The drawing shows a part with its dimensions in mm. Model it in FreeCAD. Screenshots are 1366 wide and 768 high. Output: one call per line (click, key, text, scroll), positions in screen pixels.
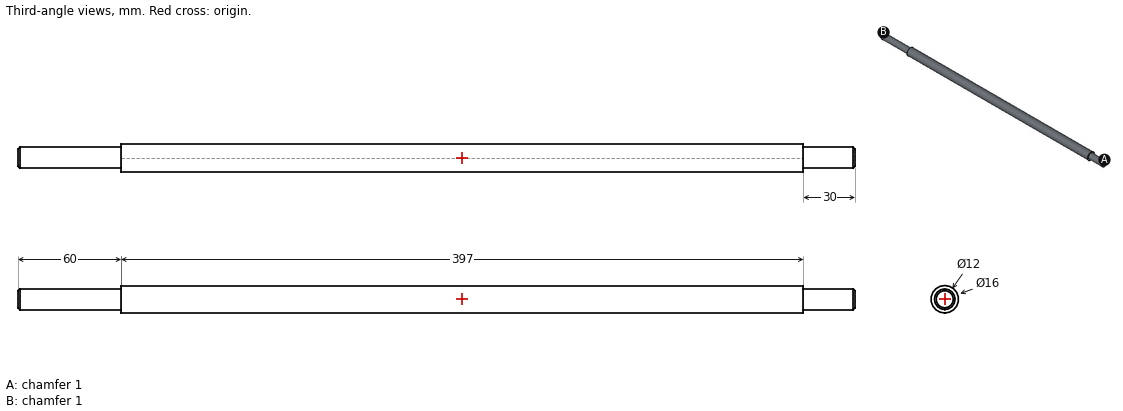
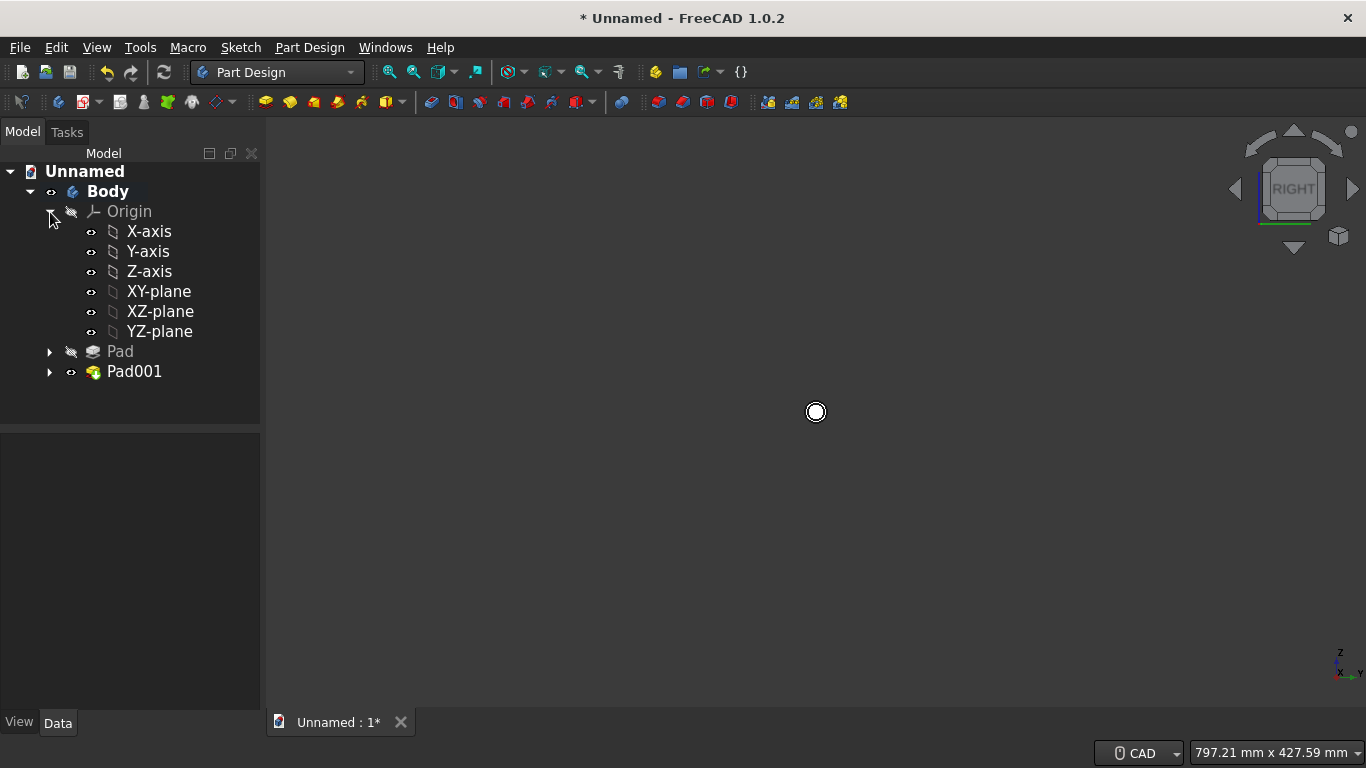
click(136, 332)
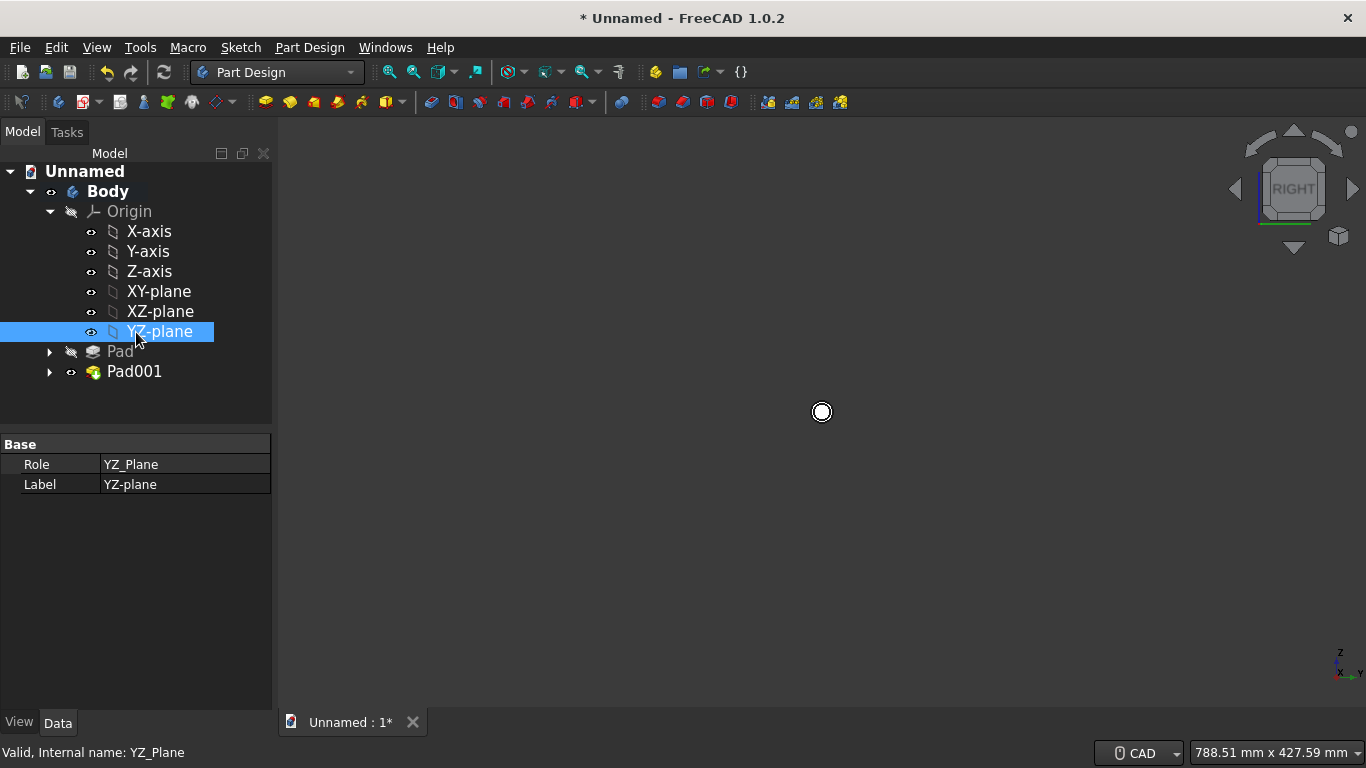
click(216, 102)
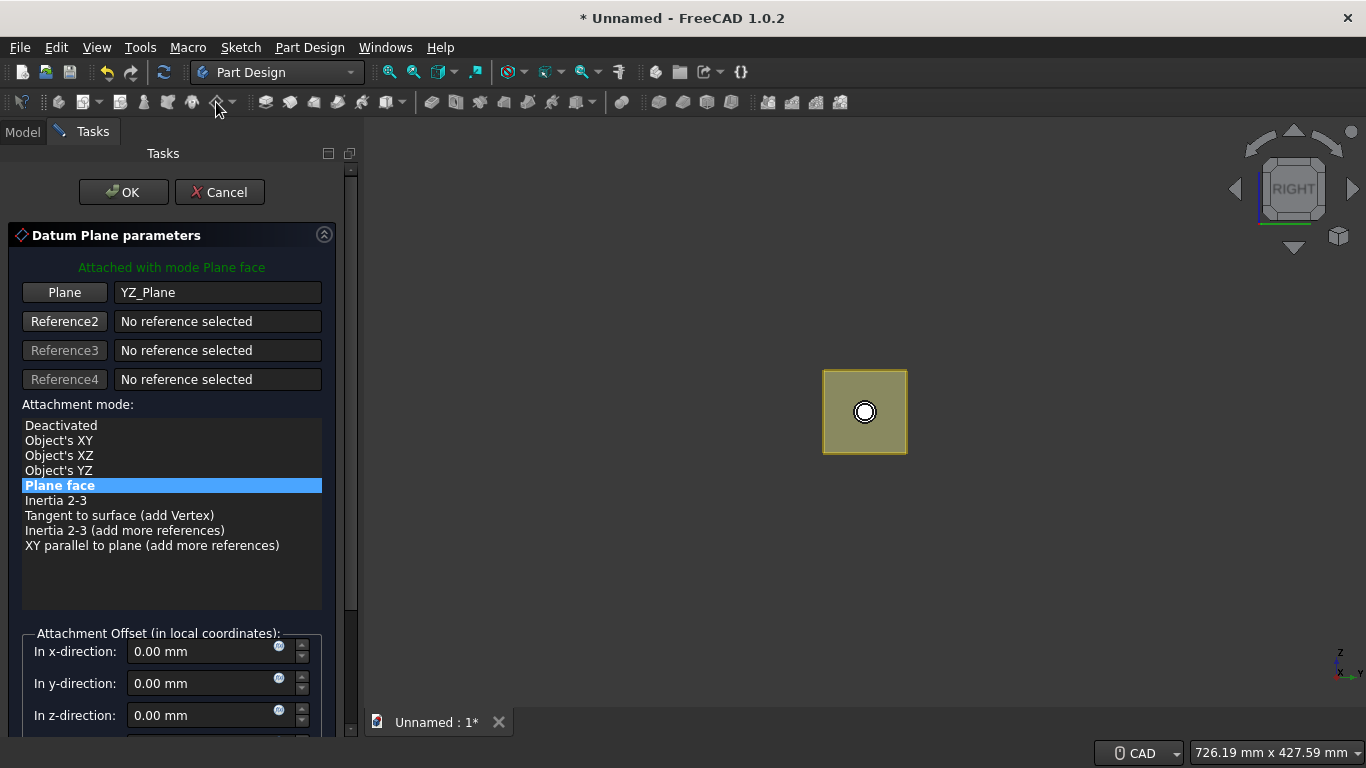
triple_click(210, 715)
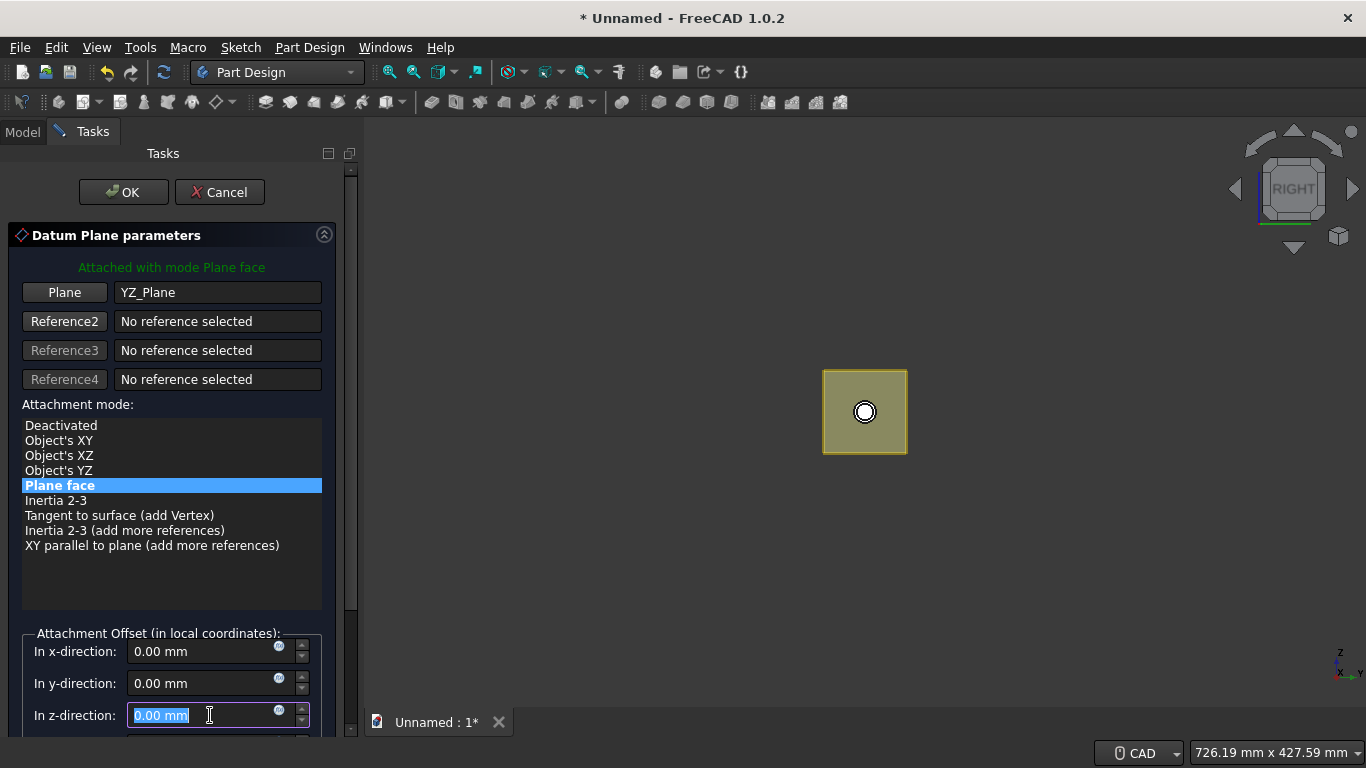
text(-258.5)
key(Tab)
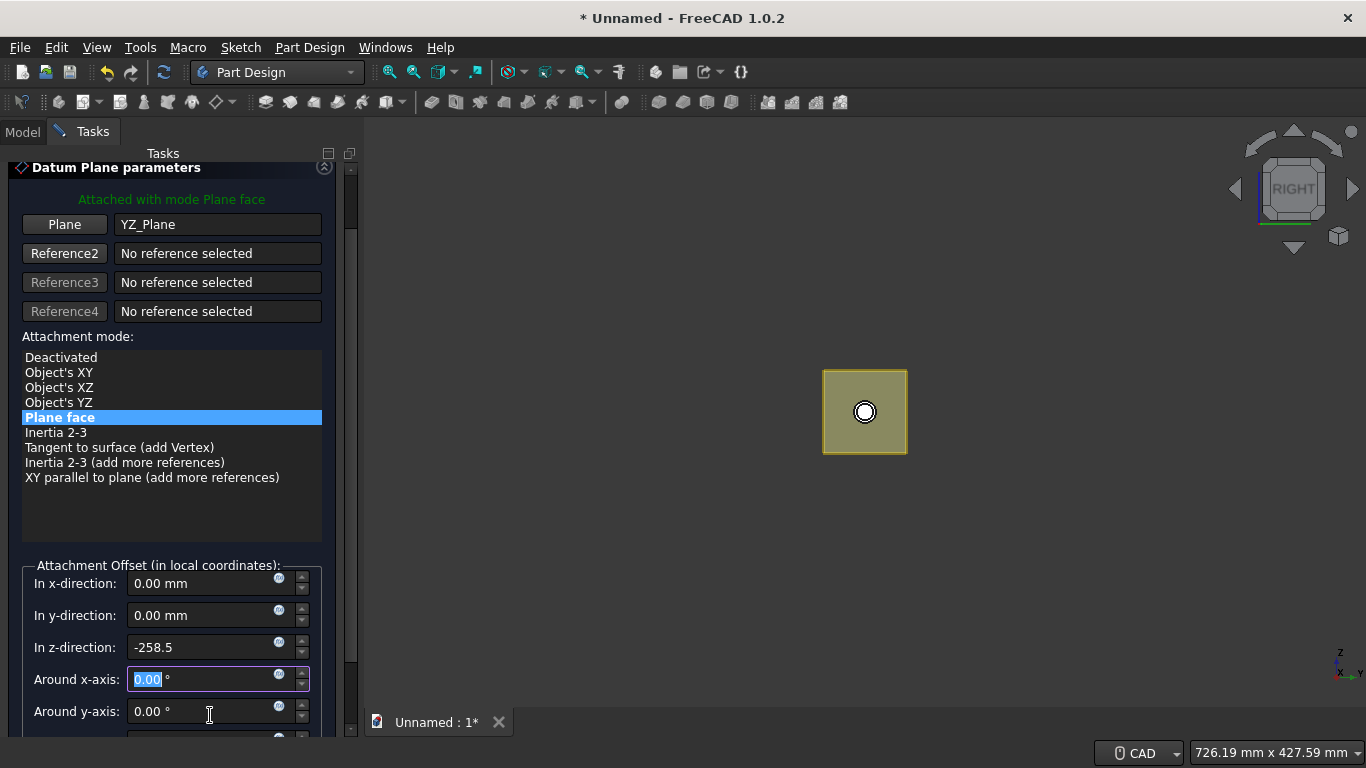
scroll(351, 450, up, 2)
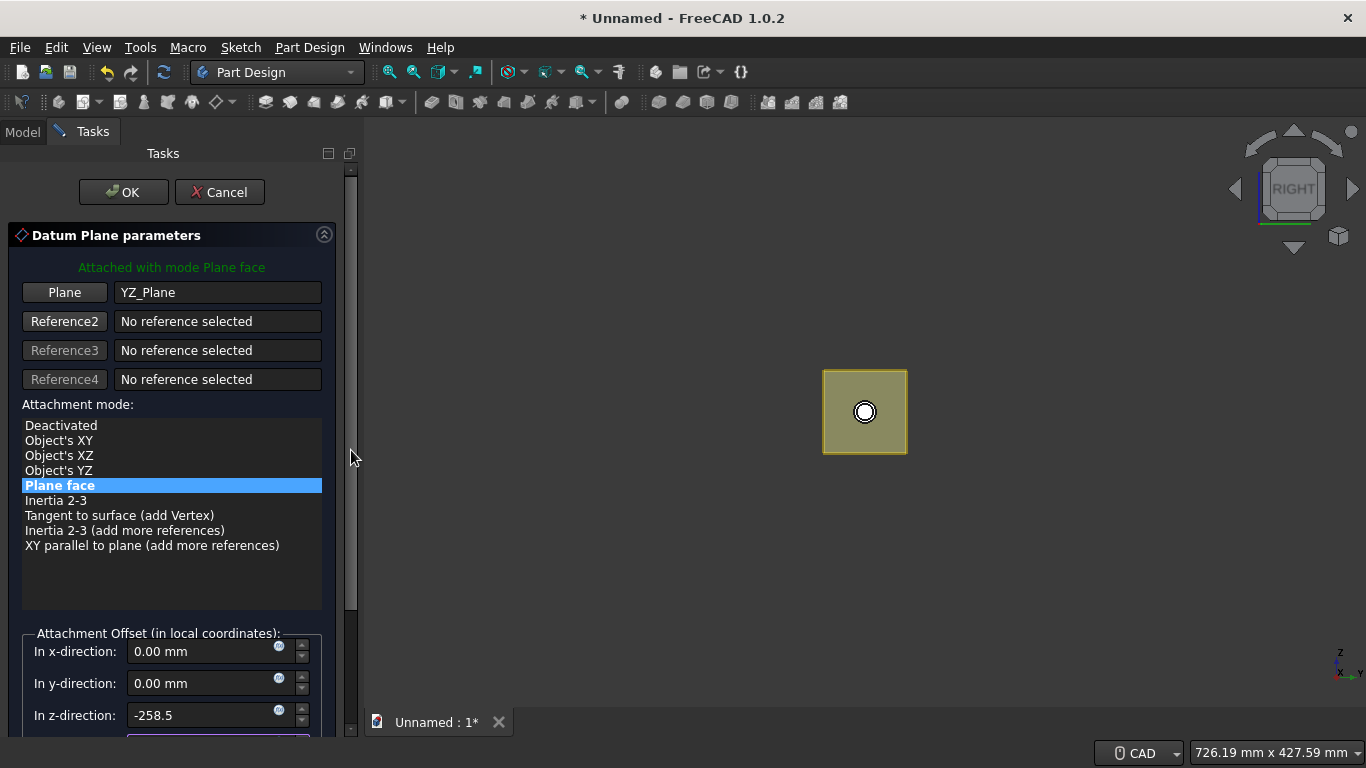
click(124, 192)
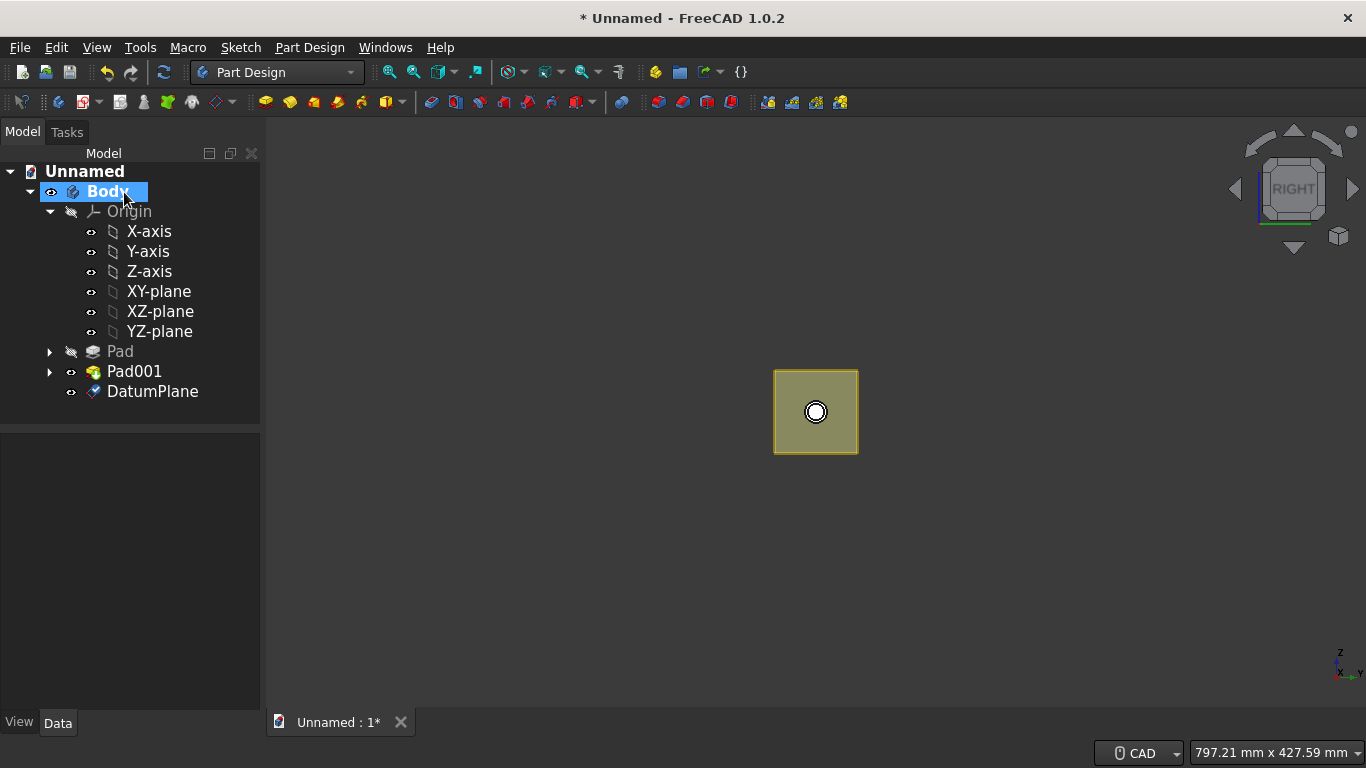
click(116, 392)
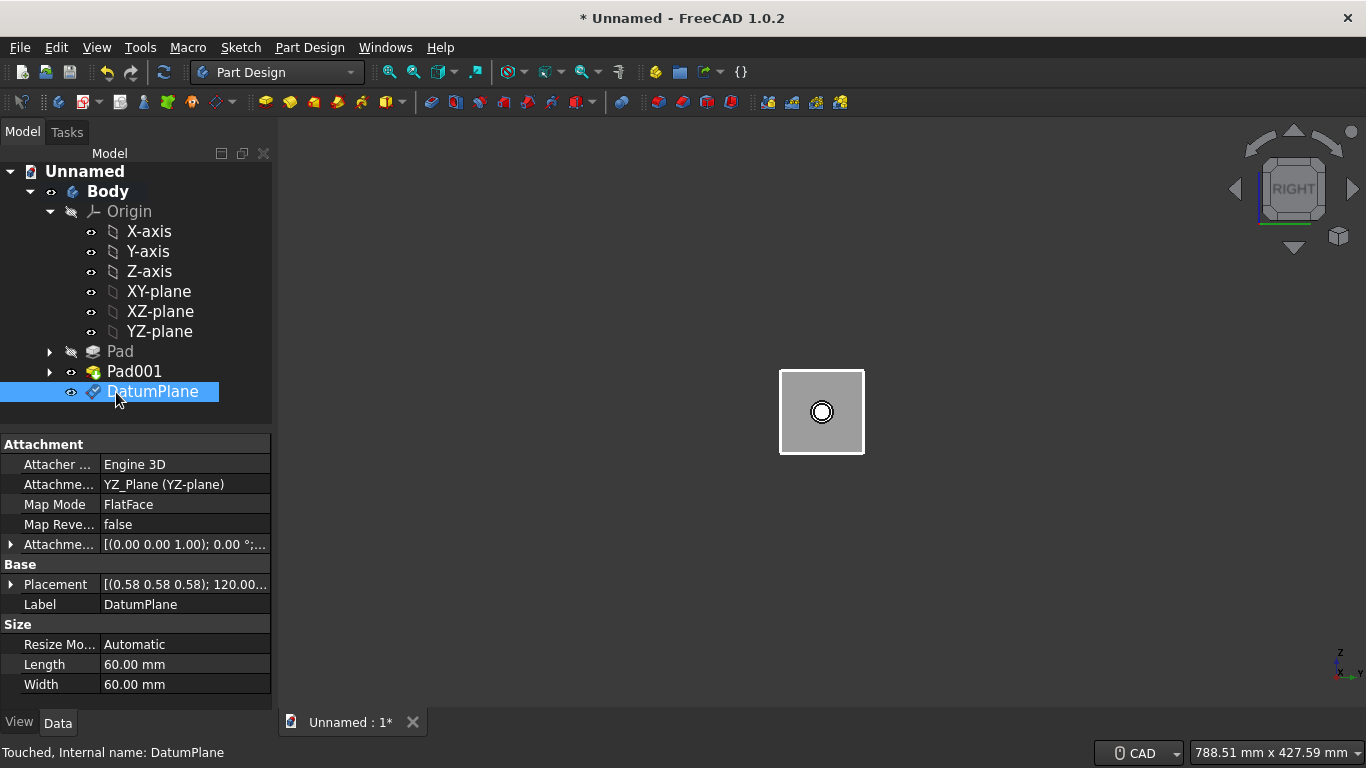
click(84, 102)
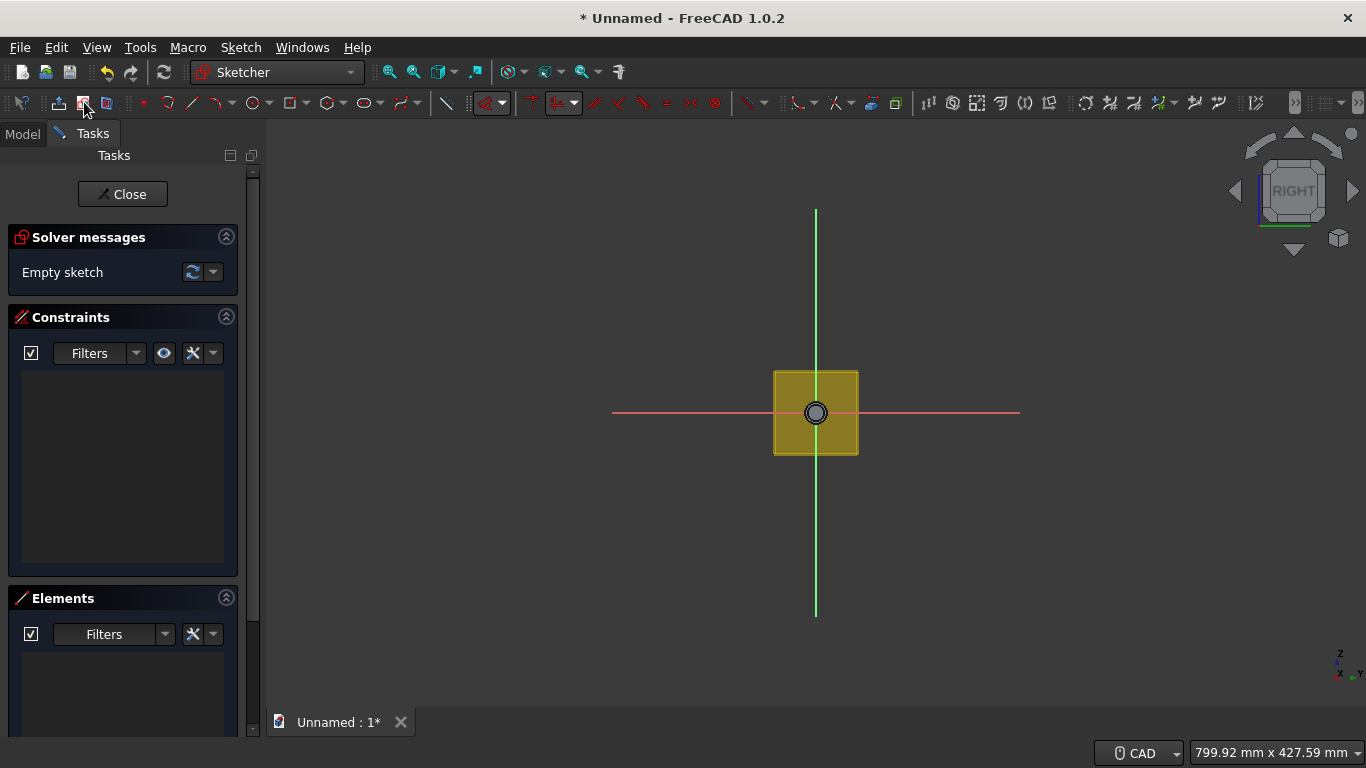
click(108, 104)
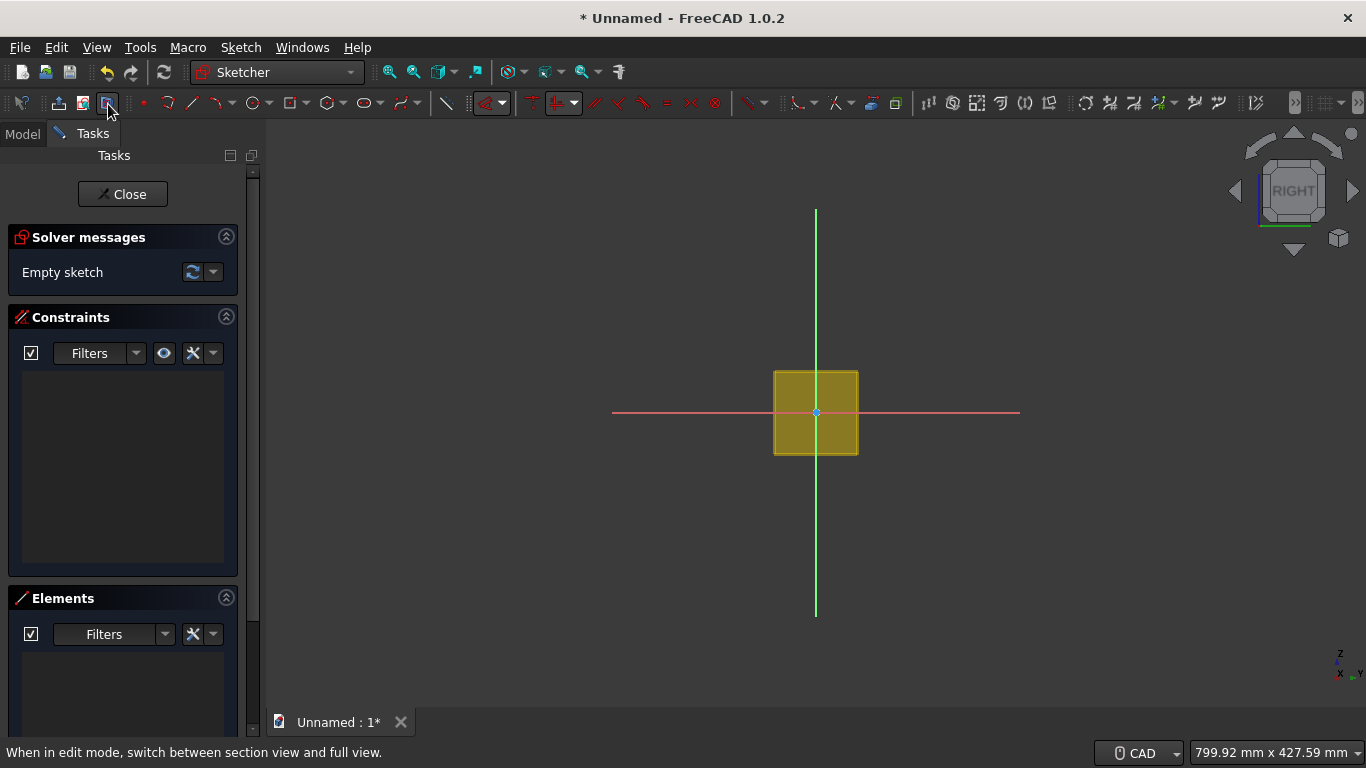
scroll(820, 413, up, 15)